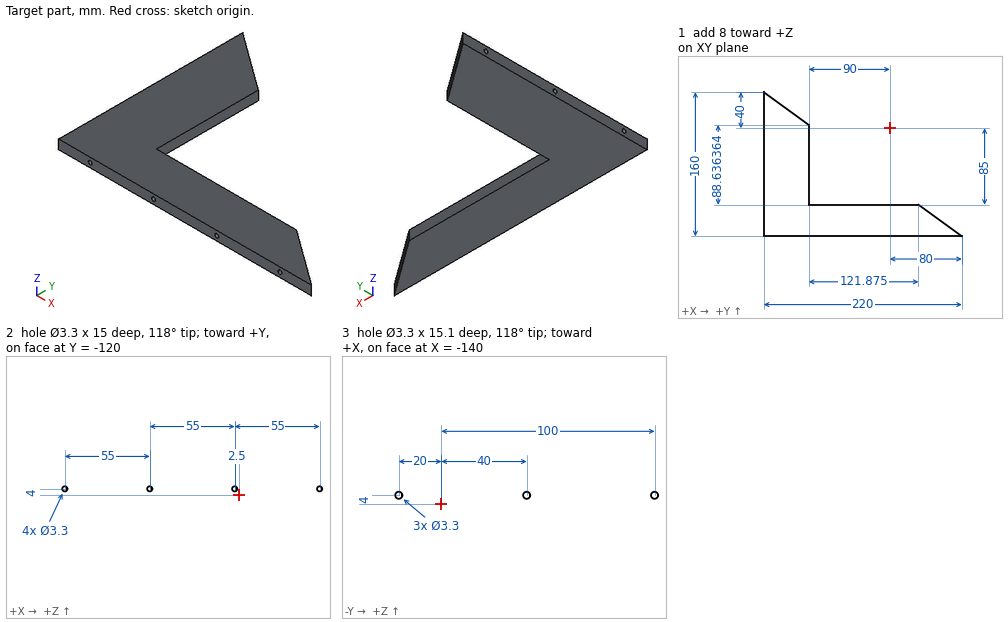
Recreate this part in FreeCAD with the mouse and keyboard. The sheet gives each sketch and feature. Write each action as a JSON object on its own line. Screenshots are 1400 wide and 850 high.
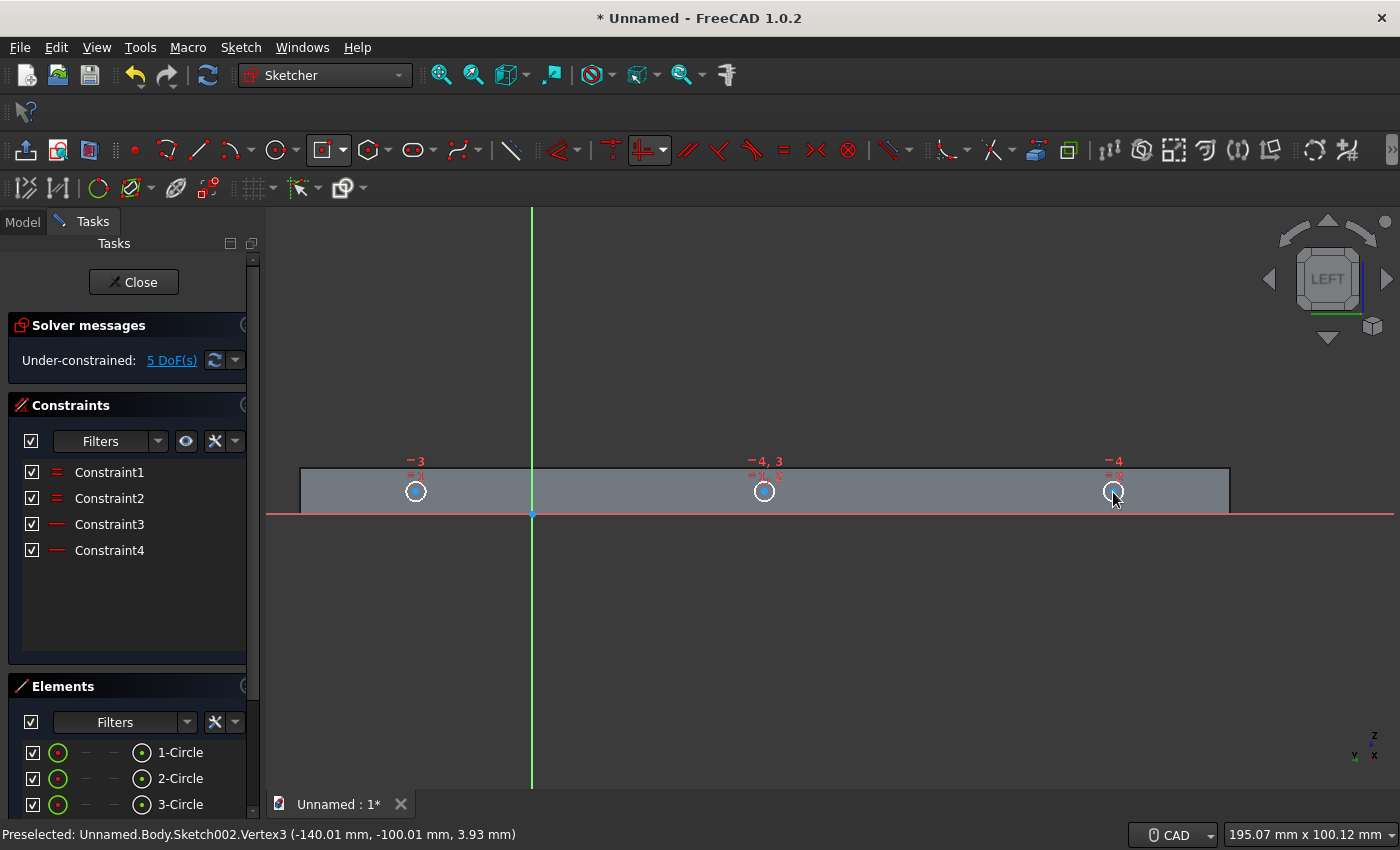
{"action": "left_click", "coordinate": [558, 150]}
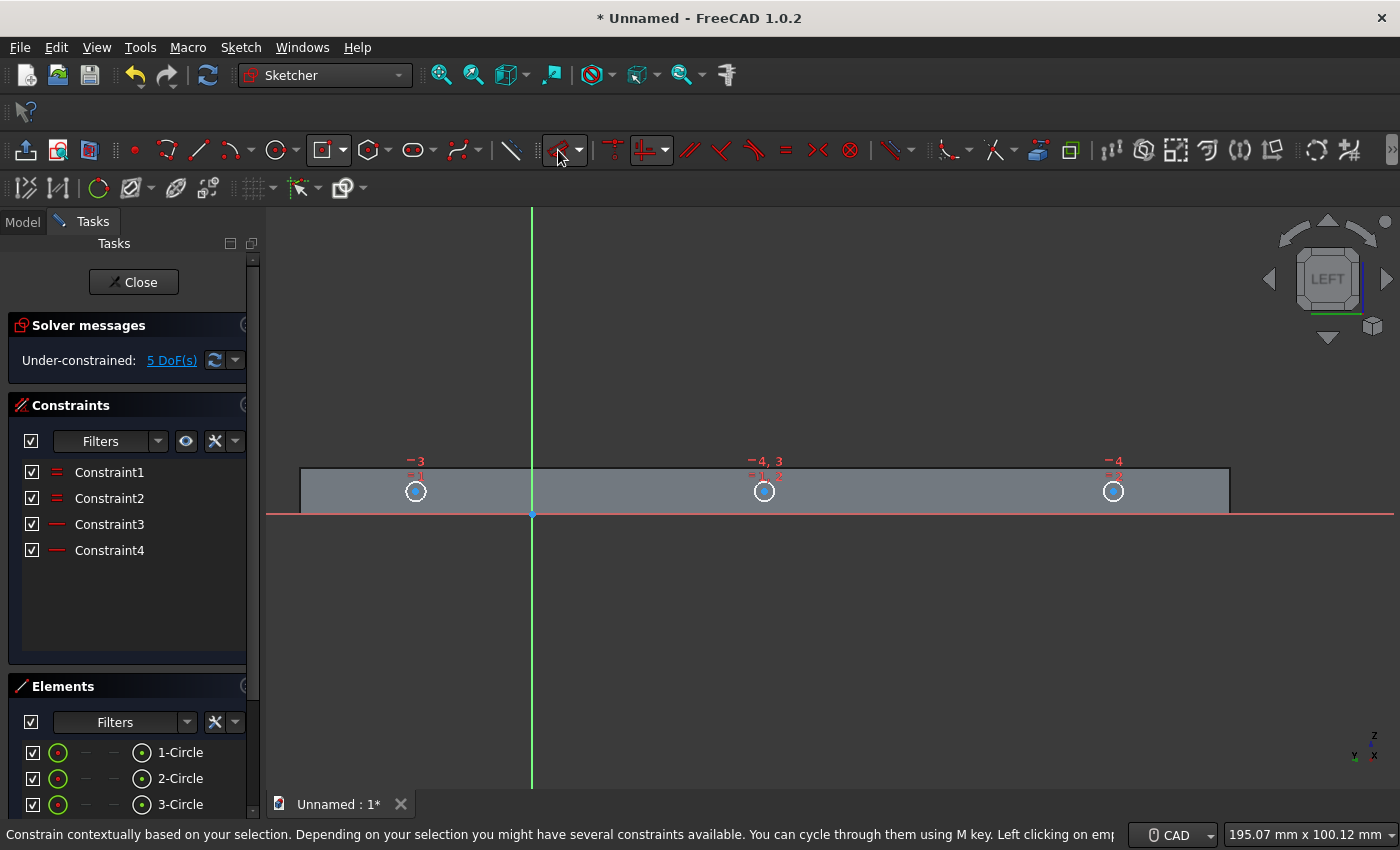
{"action": "scroll", "coordinate": [423, 485], "scroll_direction": "up", "scroll_amount": 4}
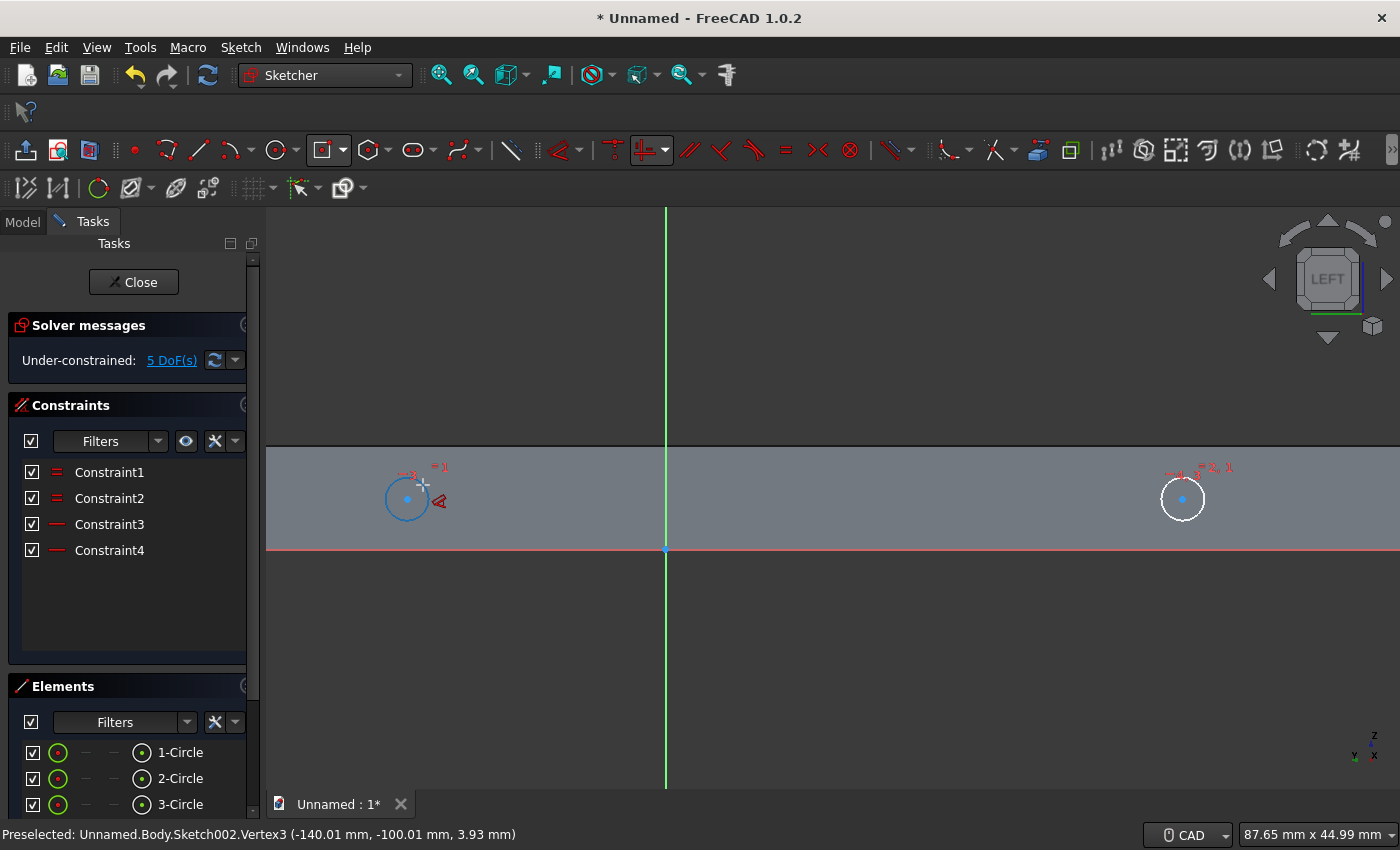
{"action": "left_click", "coordinate": [422, 484]}
{"action": "left_click", "coordinate": [444, 461]}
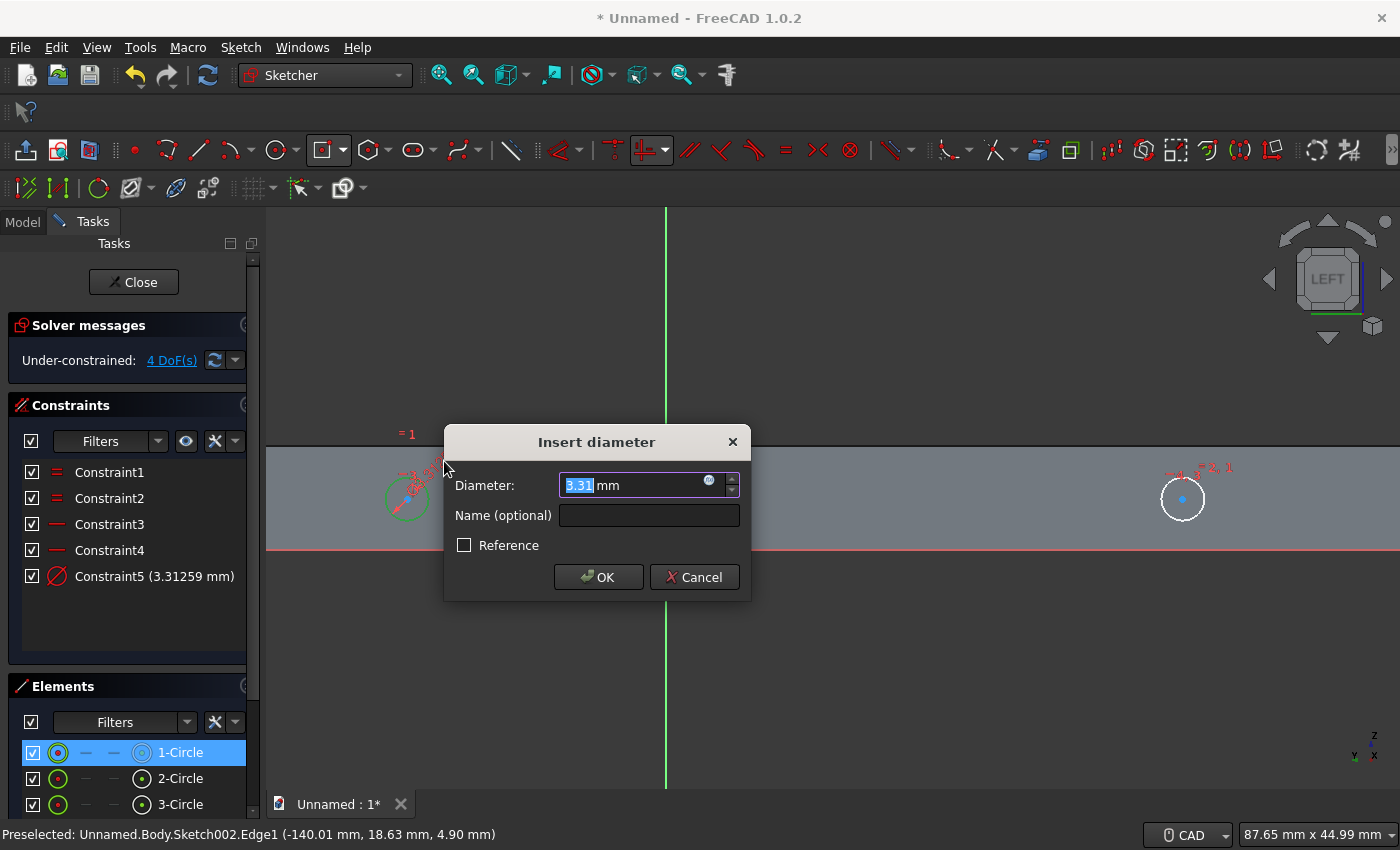
{"action": "type", "text": "3.3"}
{"action": "key", "text": "Return"}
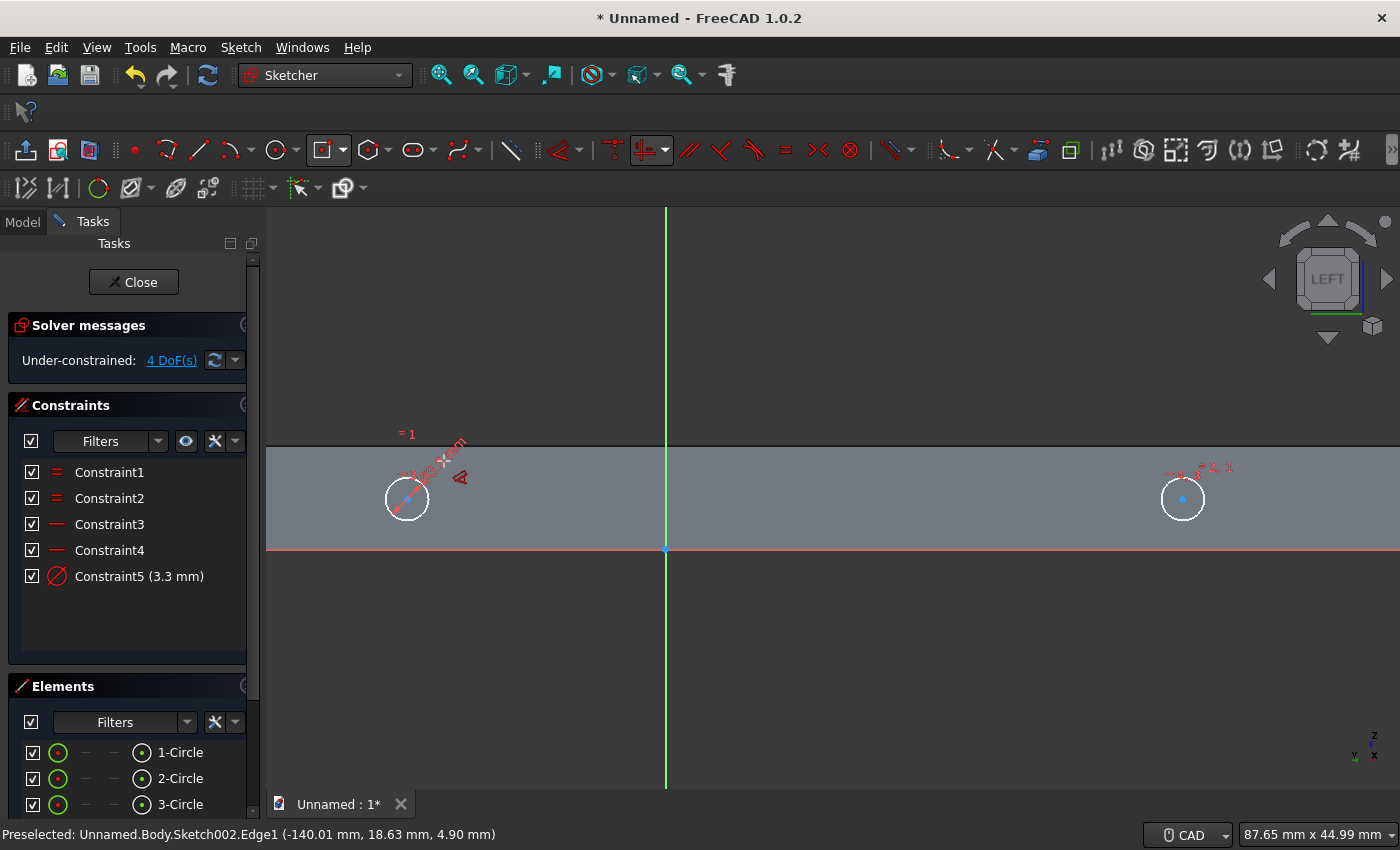
{"action": "left_click", "coordinate": [407, 499]}
{"action": "left_click", "coordinate": [373, 525]}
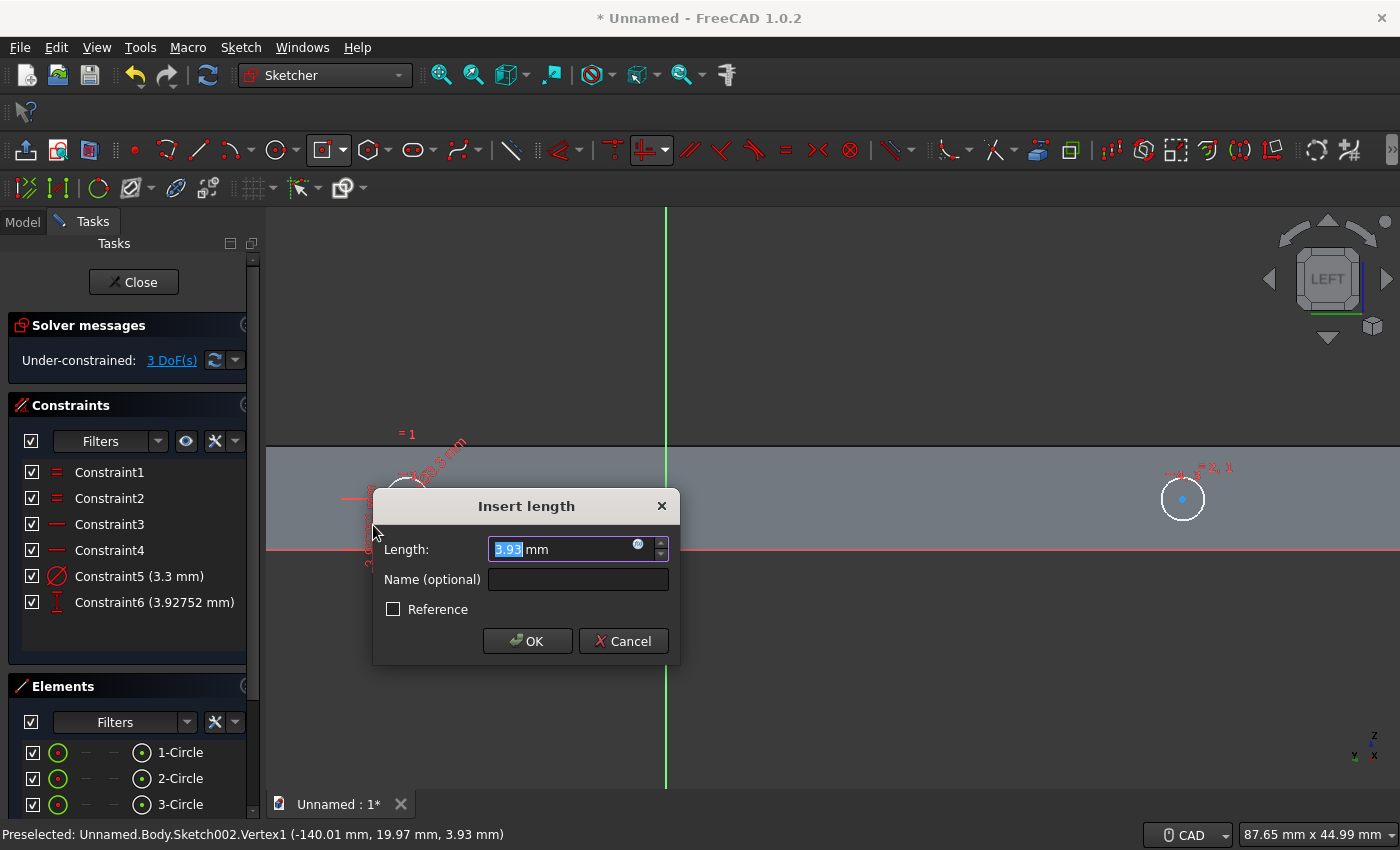
{"action": "type", "text": "4"}
{"action": "key", "text": "Return"}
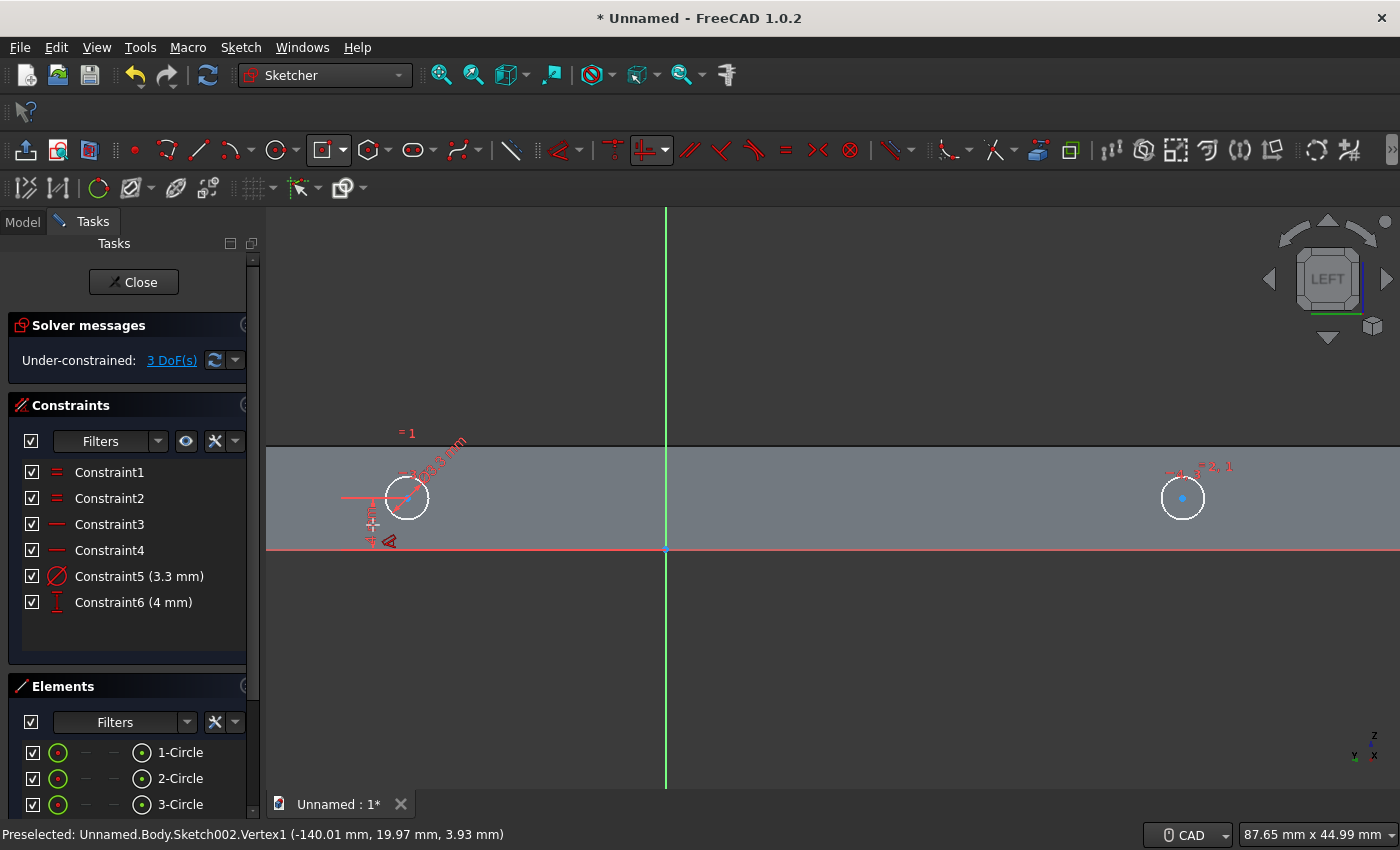
{"action": "left_click", "coordinate": [407, 498]}
{"action": "left_click", "coordinate": [536, 584]}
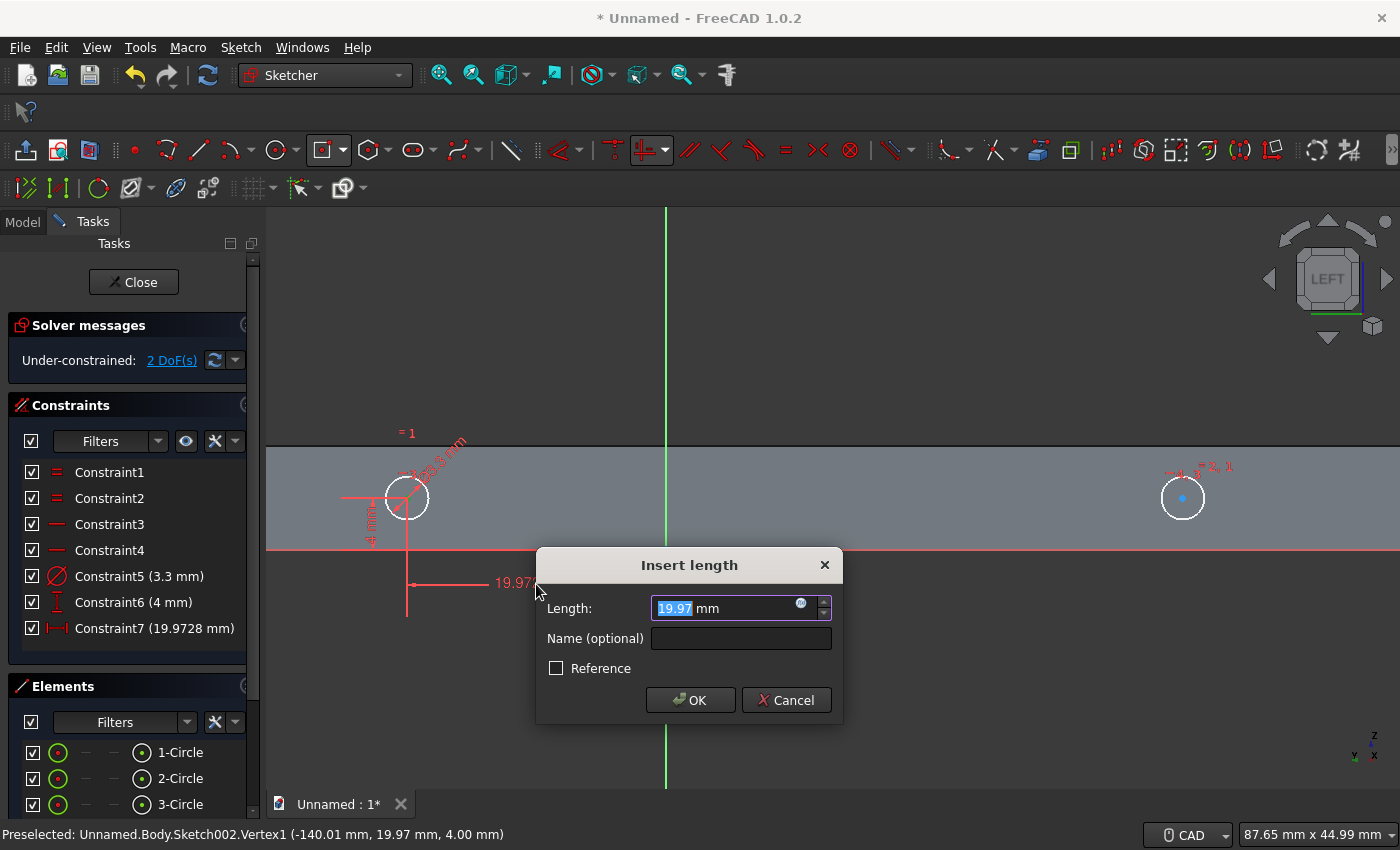
{"action": "type", "text": "20"}
{"action": "key", "text": "Return"}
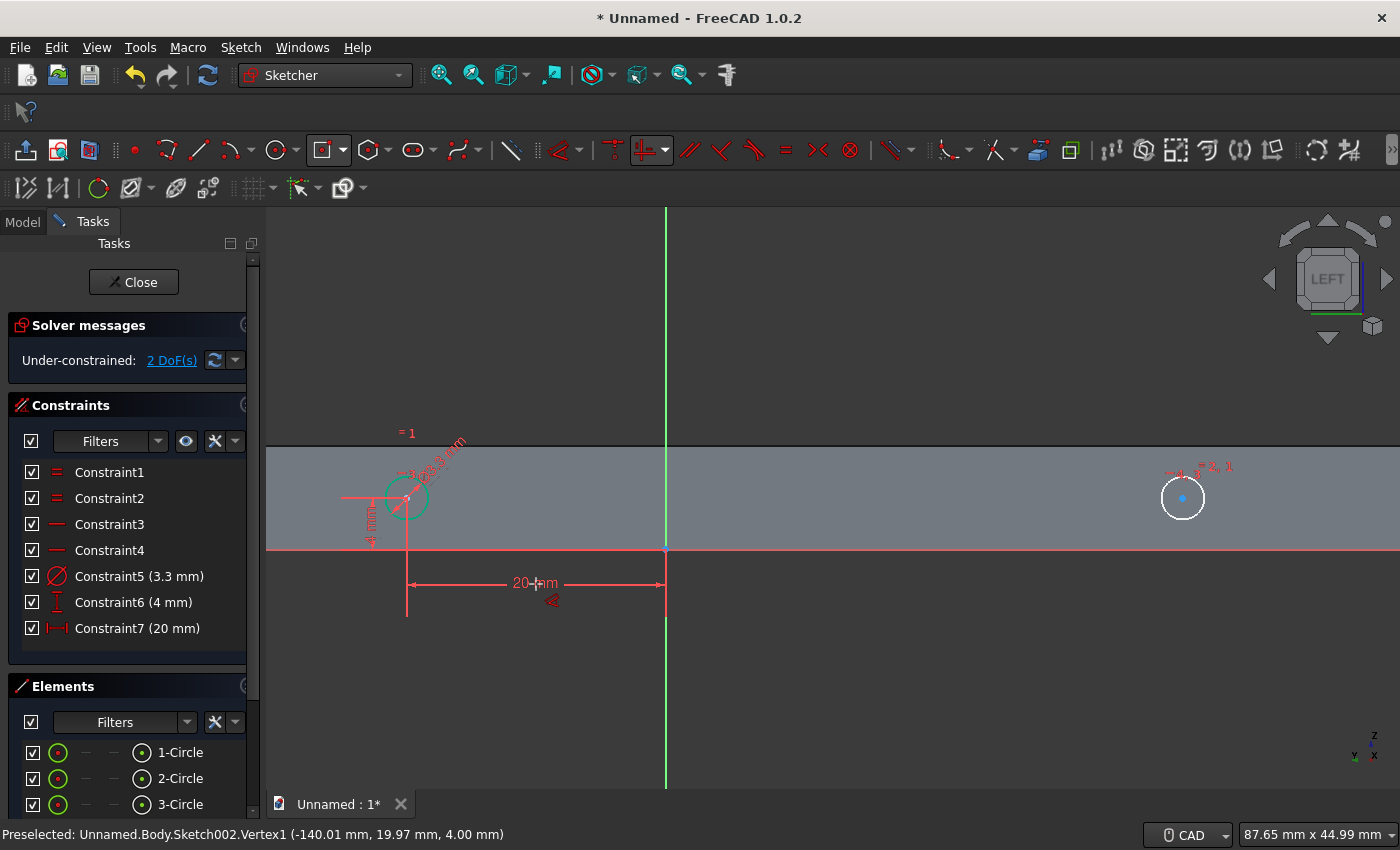
{"action": "left_click", "coordinate": [1183, 498]}
{"action": "left_click", "coordinate": [924, 584]}